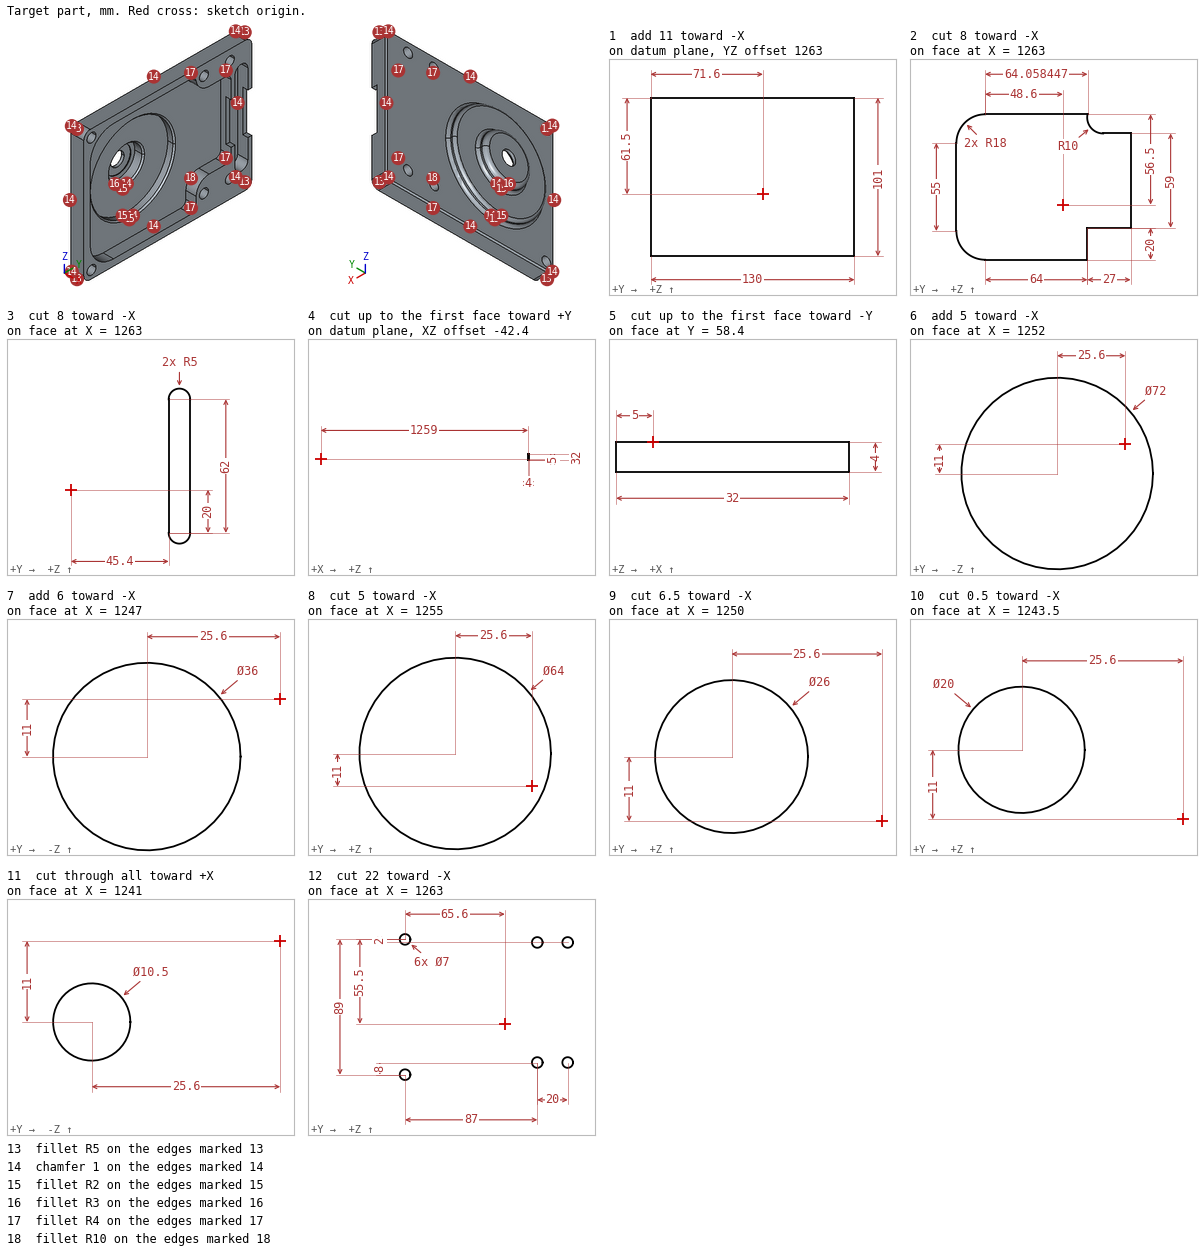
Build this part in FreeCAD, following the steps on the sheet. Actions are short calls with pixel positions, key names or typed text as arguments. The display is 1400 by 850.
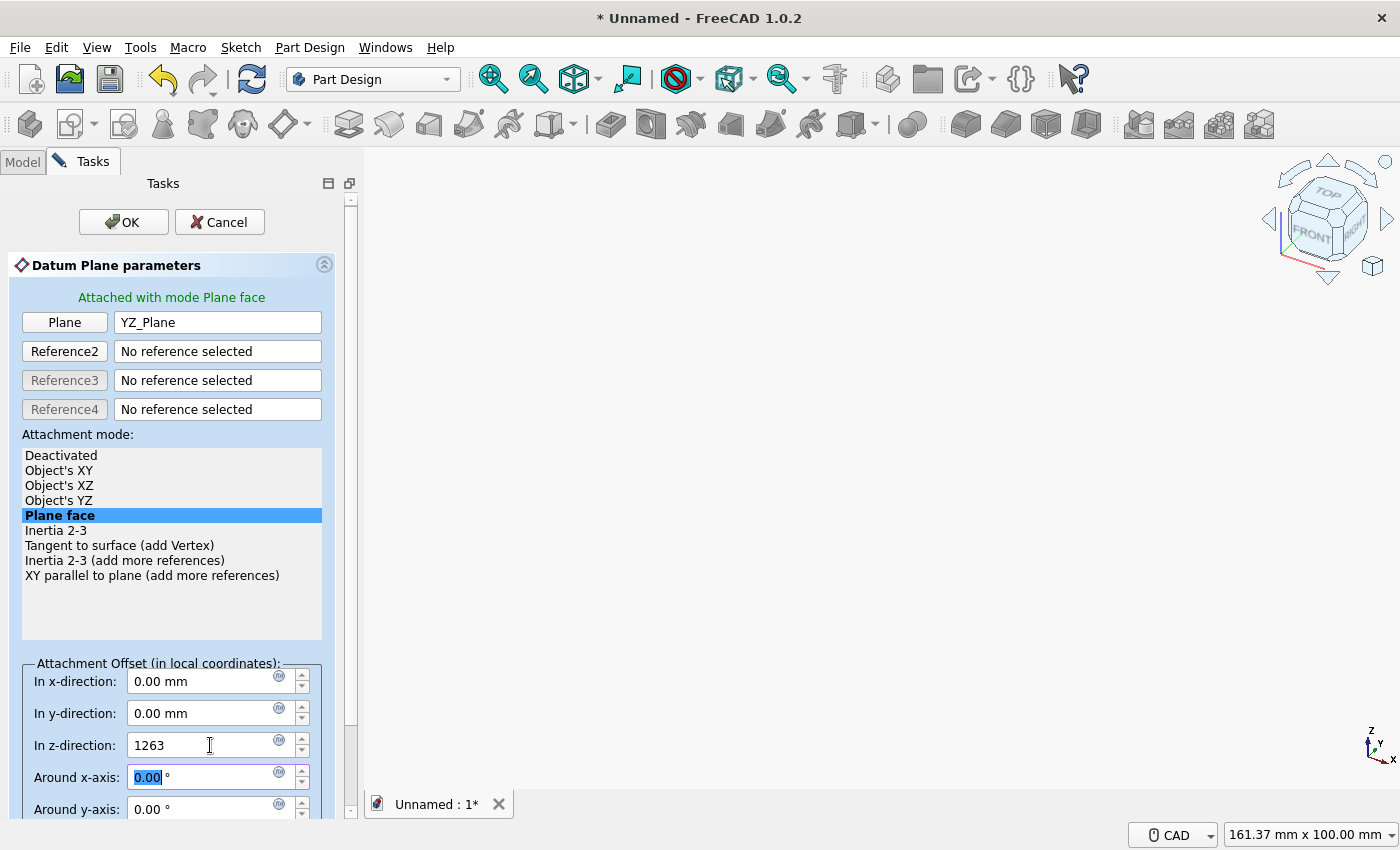
click(124, 222)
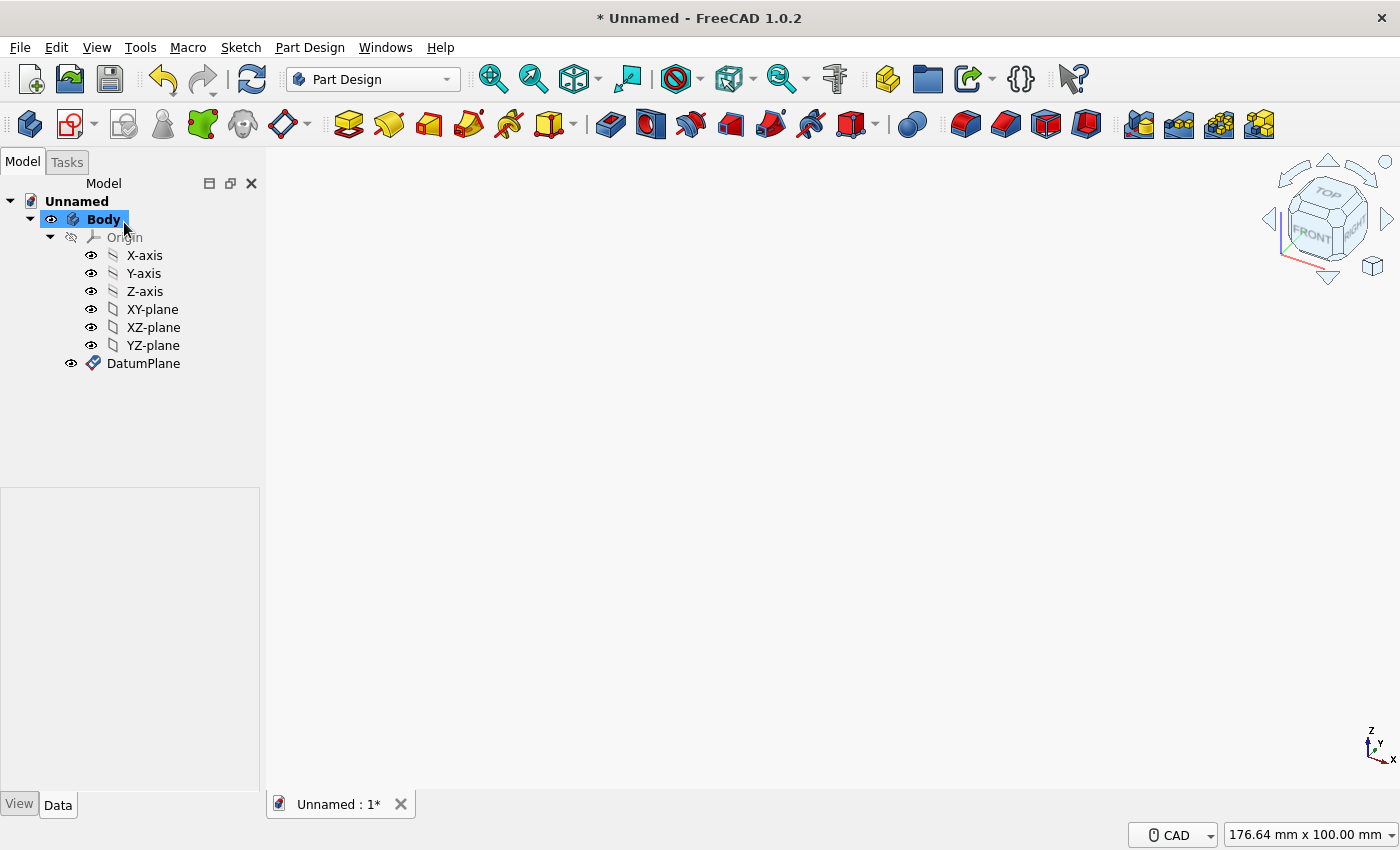
click(116, 363)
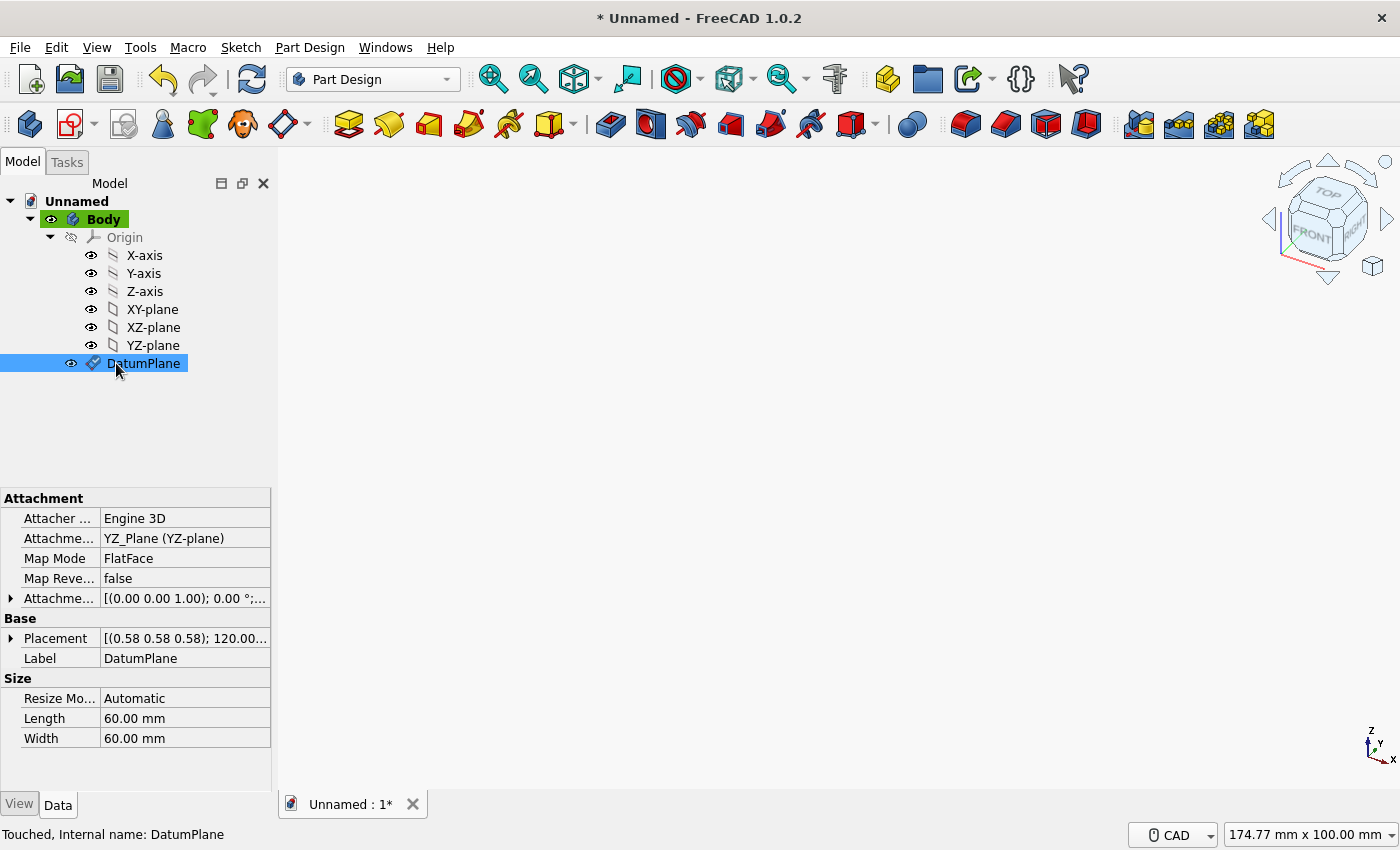
click(70, 124)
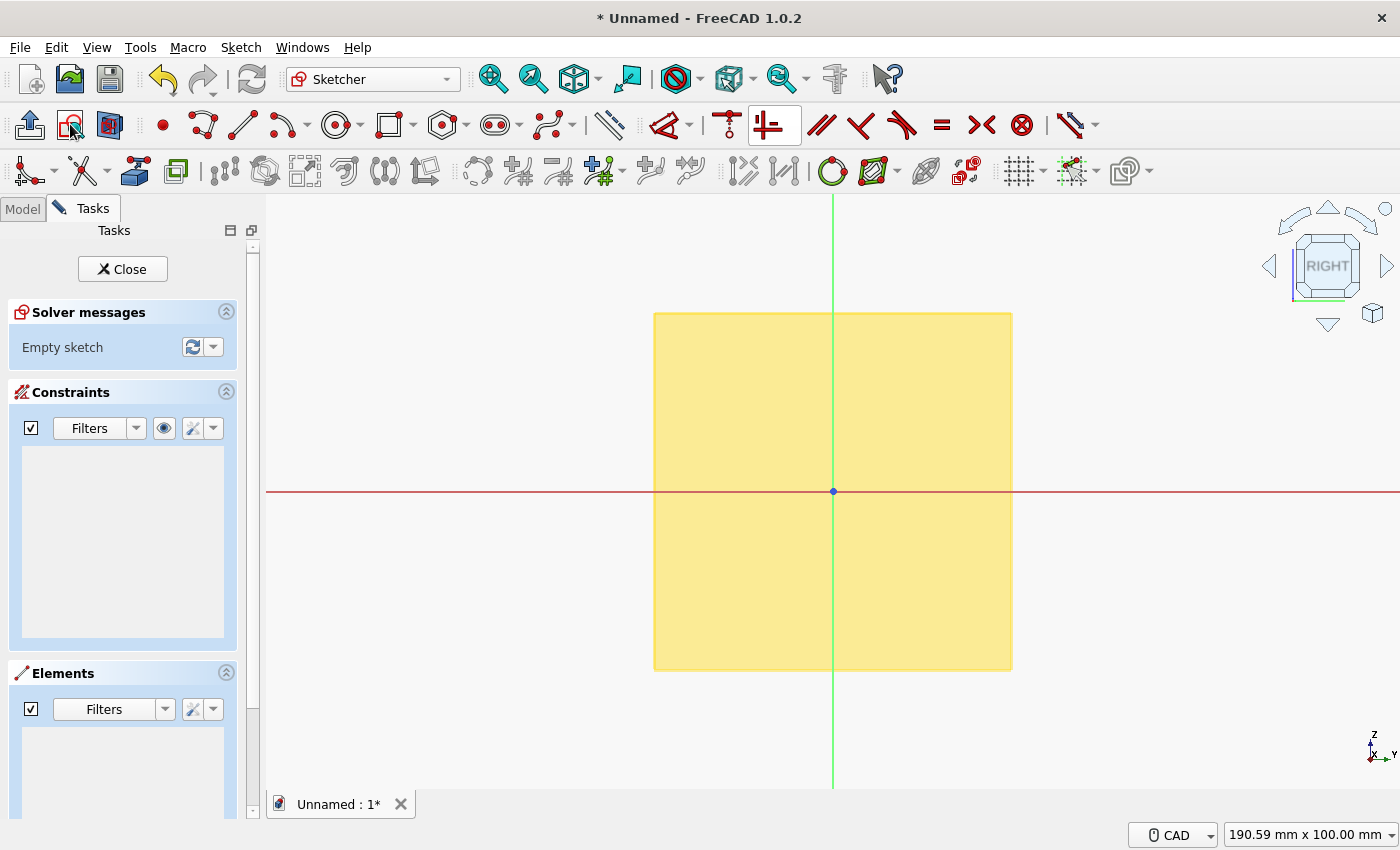
scroll(705, 625, down, 2)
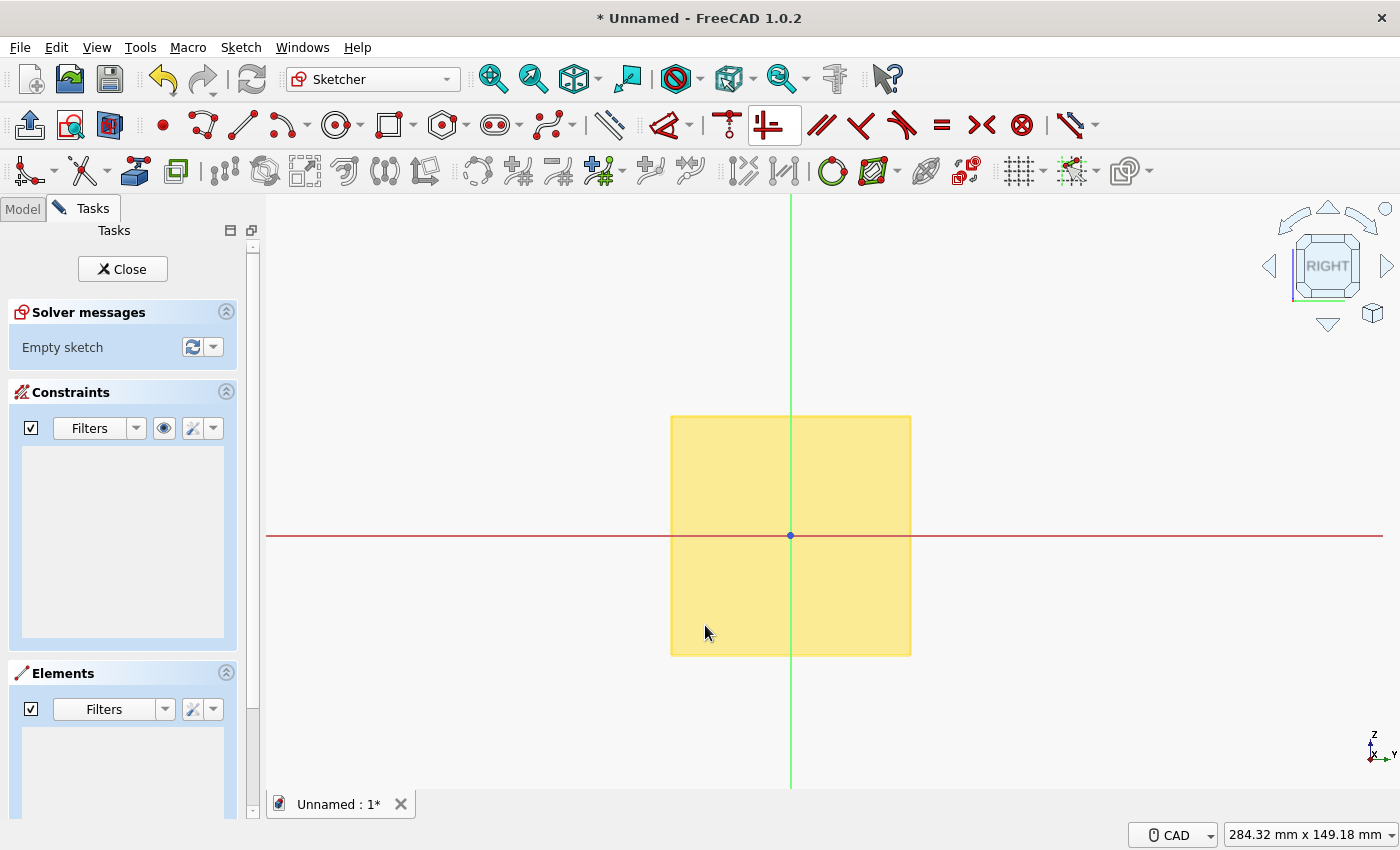
click(390, 126)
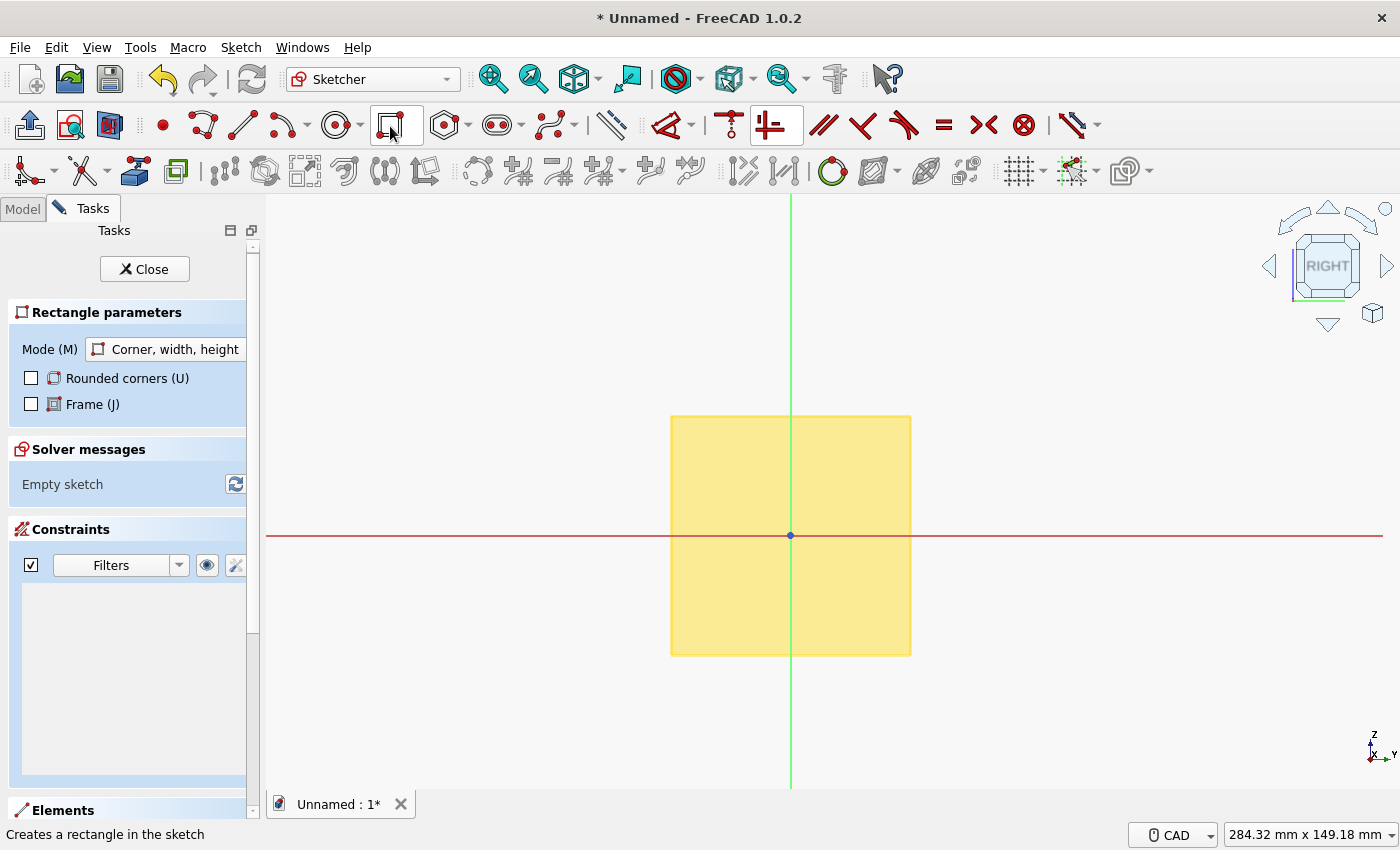
click(505, 290)
move(1024, 693)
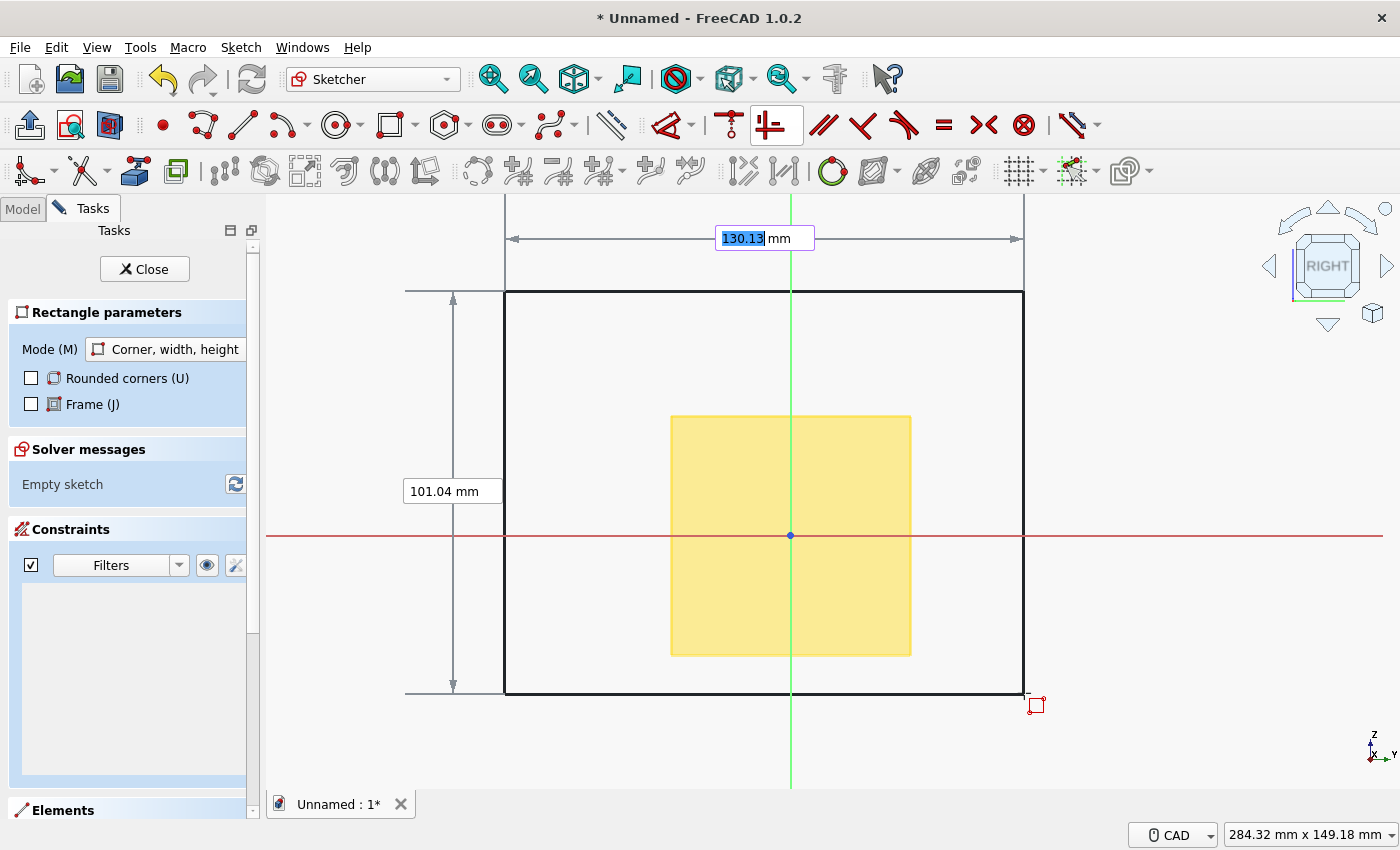
text(130)
key(Tab)
text(101)
key(Return)
key(Escape)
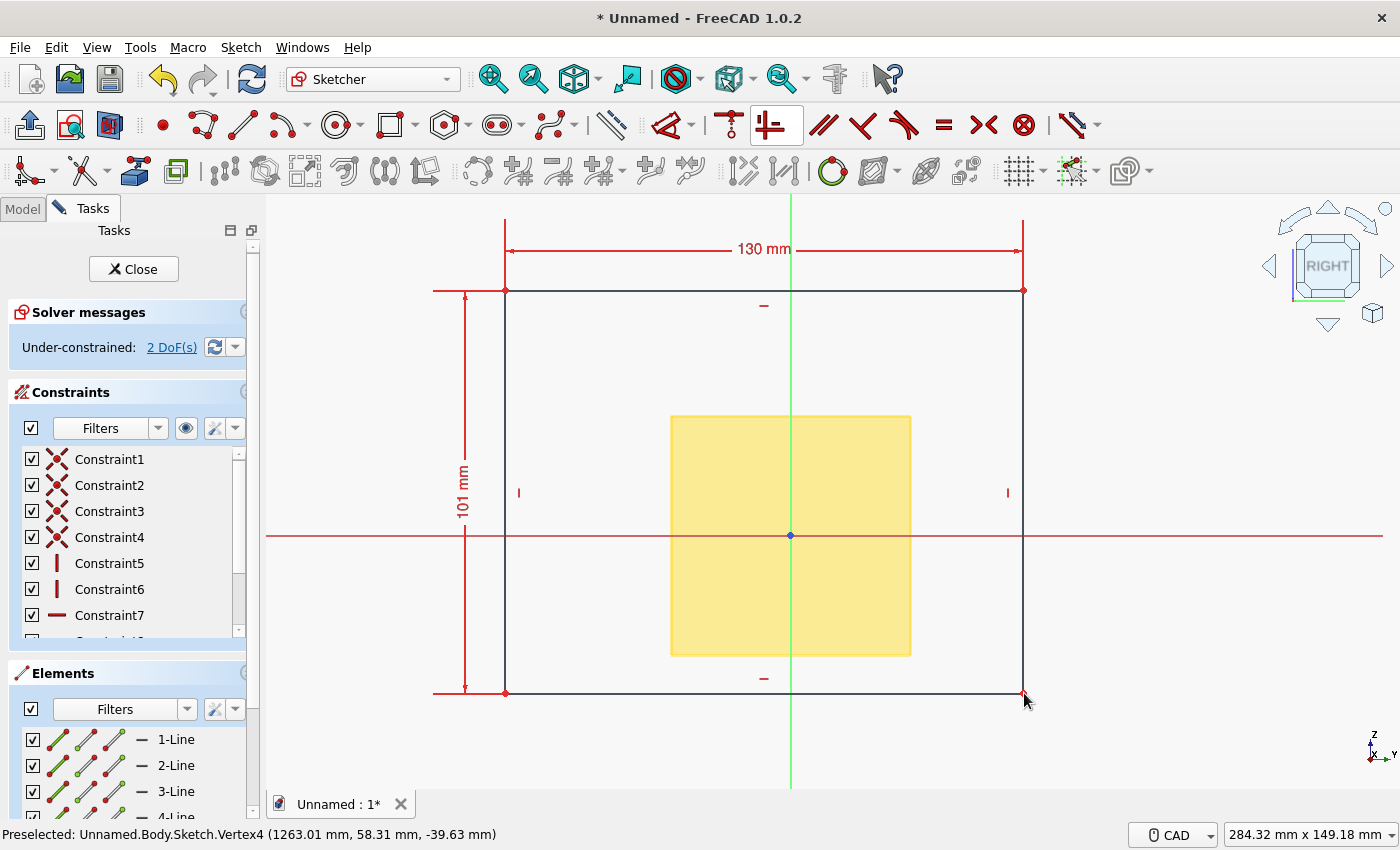
click(505, 291)